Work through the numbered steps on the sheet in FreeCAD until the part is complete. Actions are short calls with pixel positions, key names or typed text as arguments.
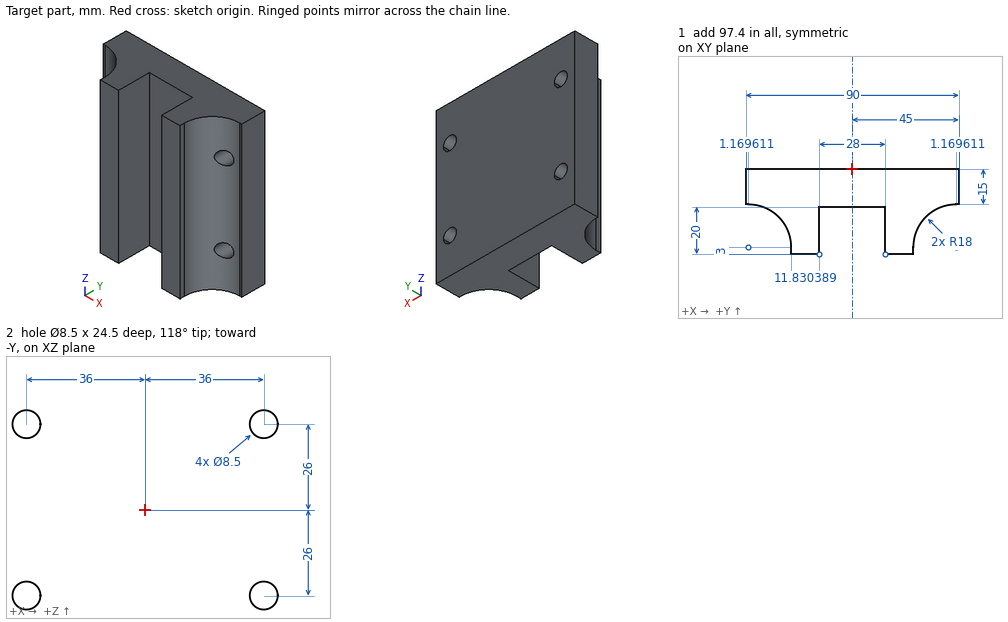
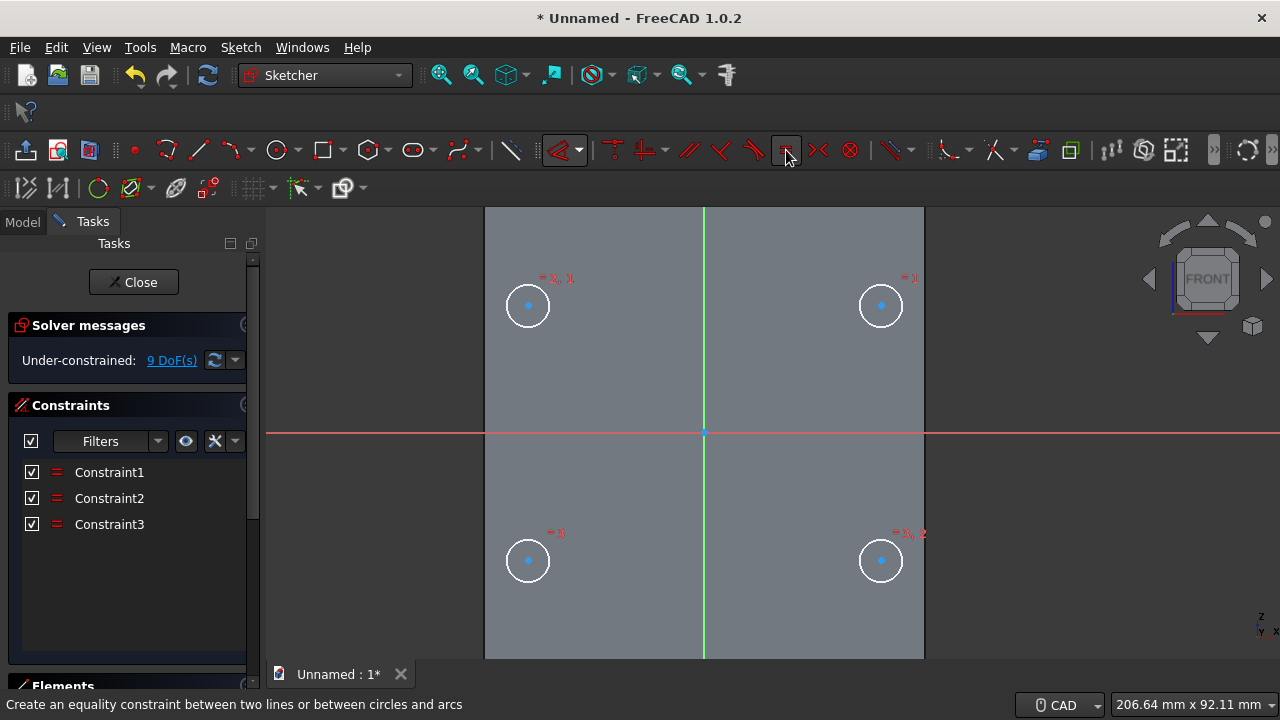
click(881, 306)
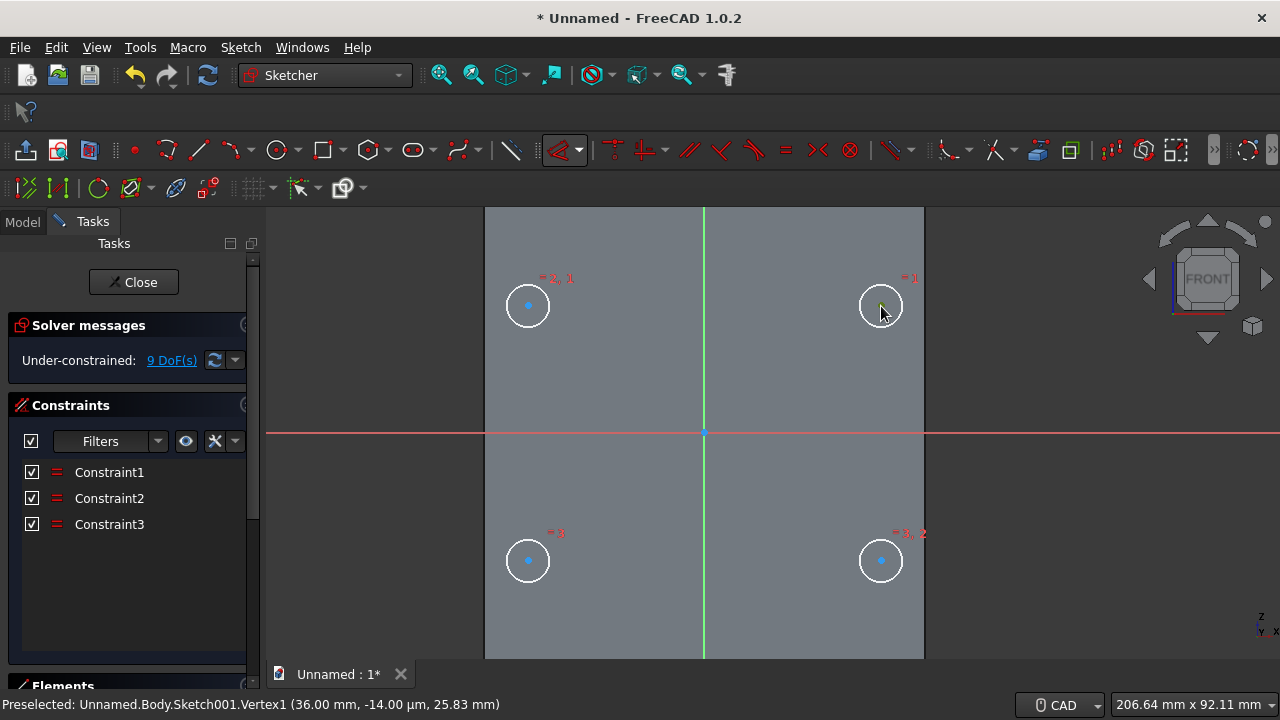
click(528, 306)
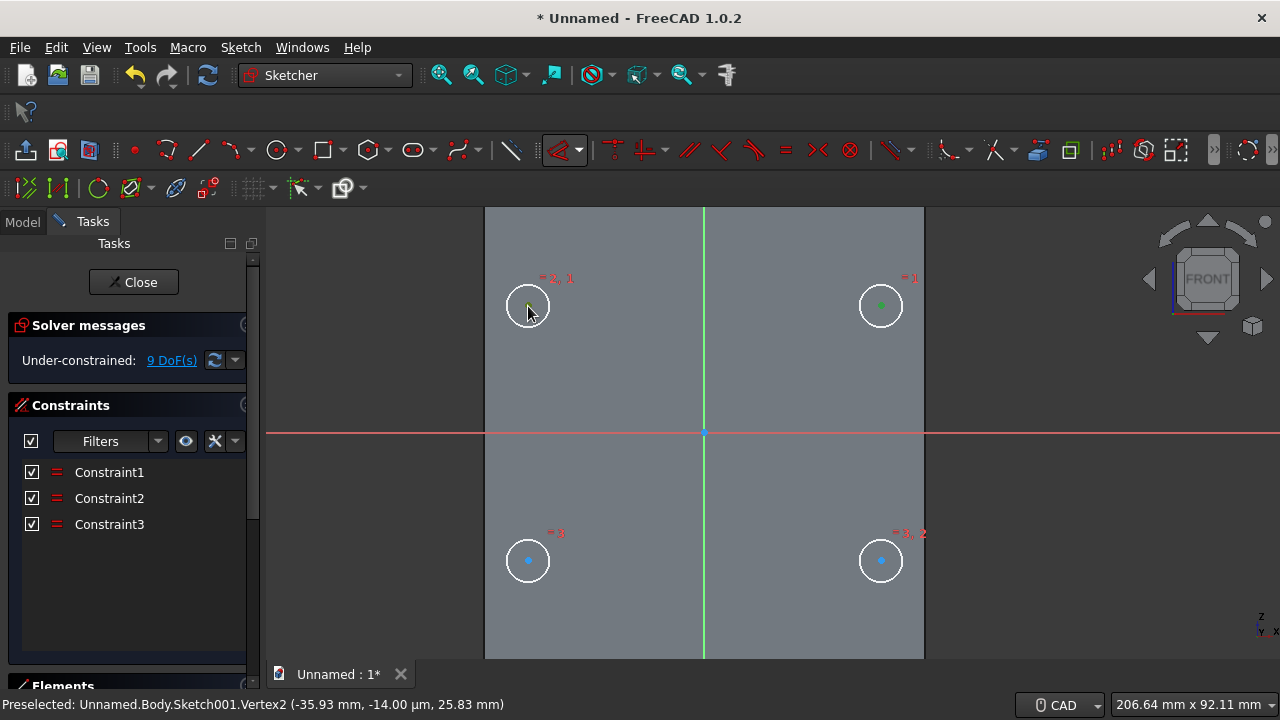
key(h)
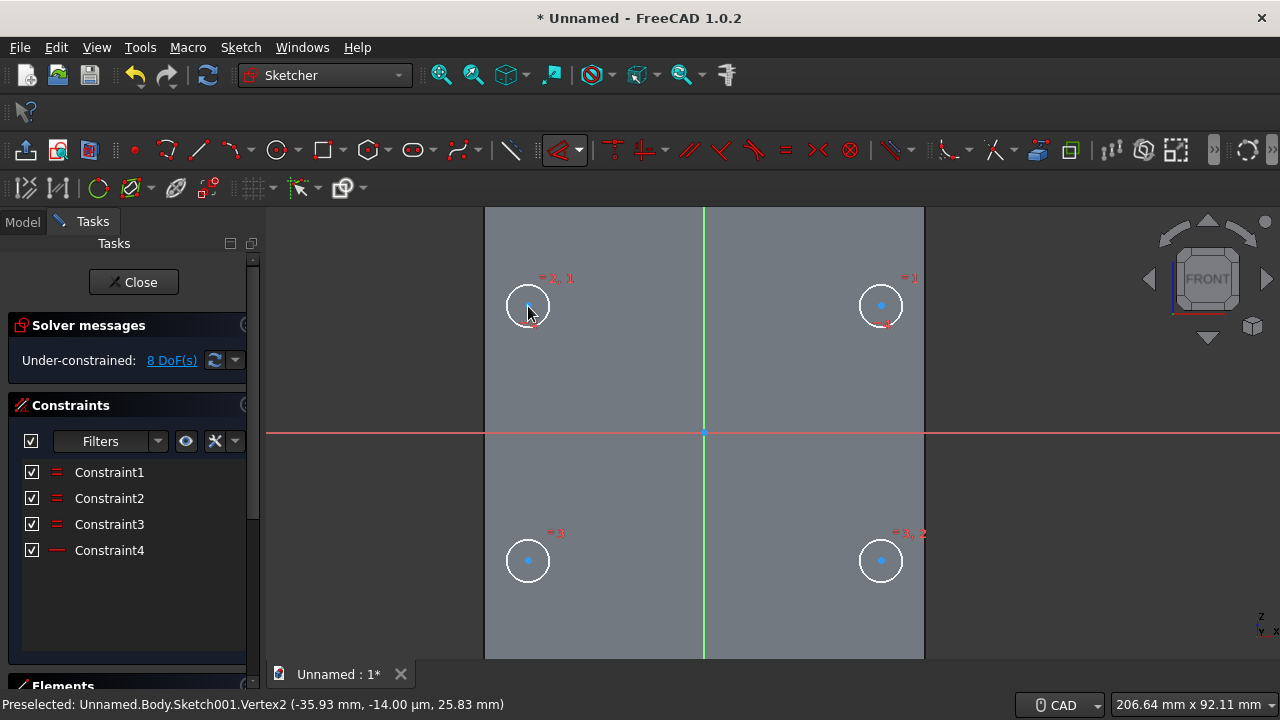
click(881, 306)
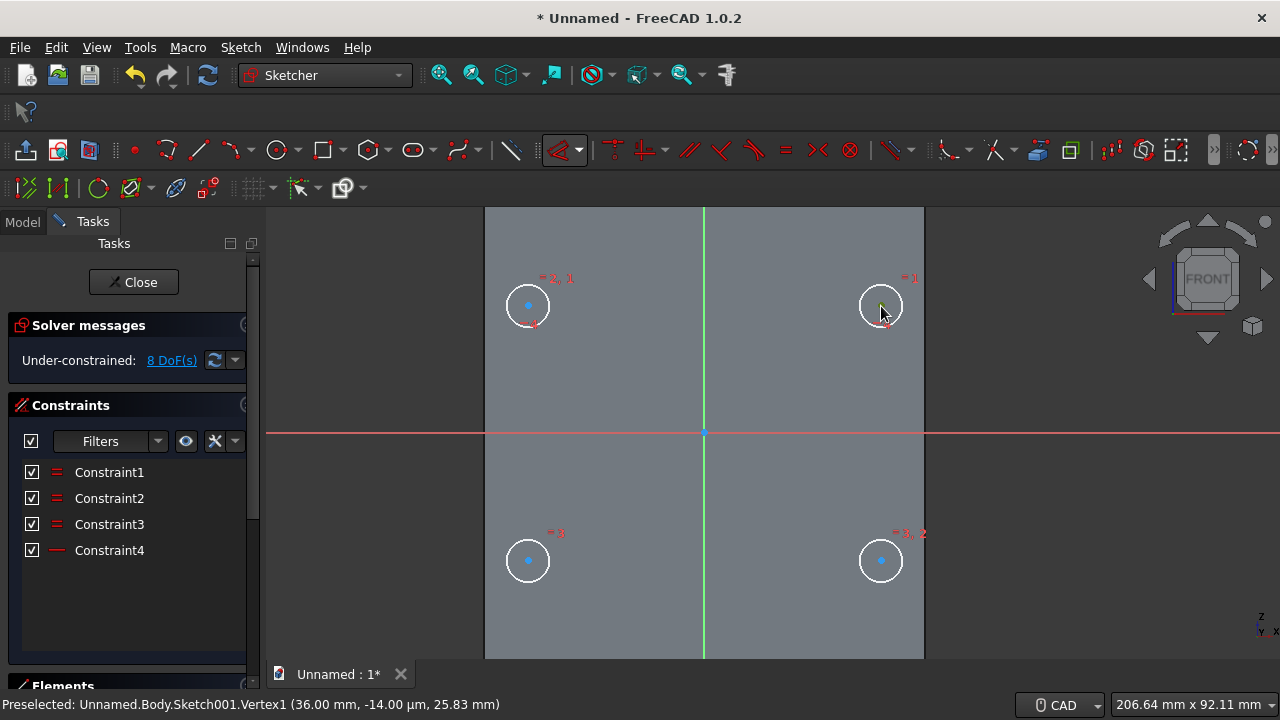
click(881, 561)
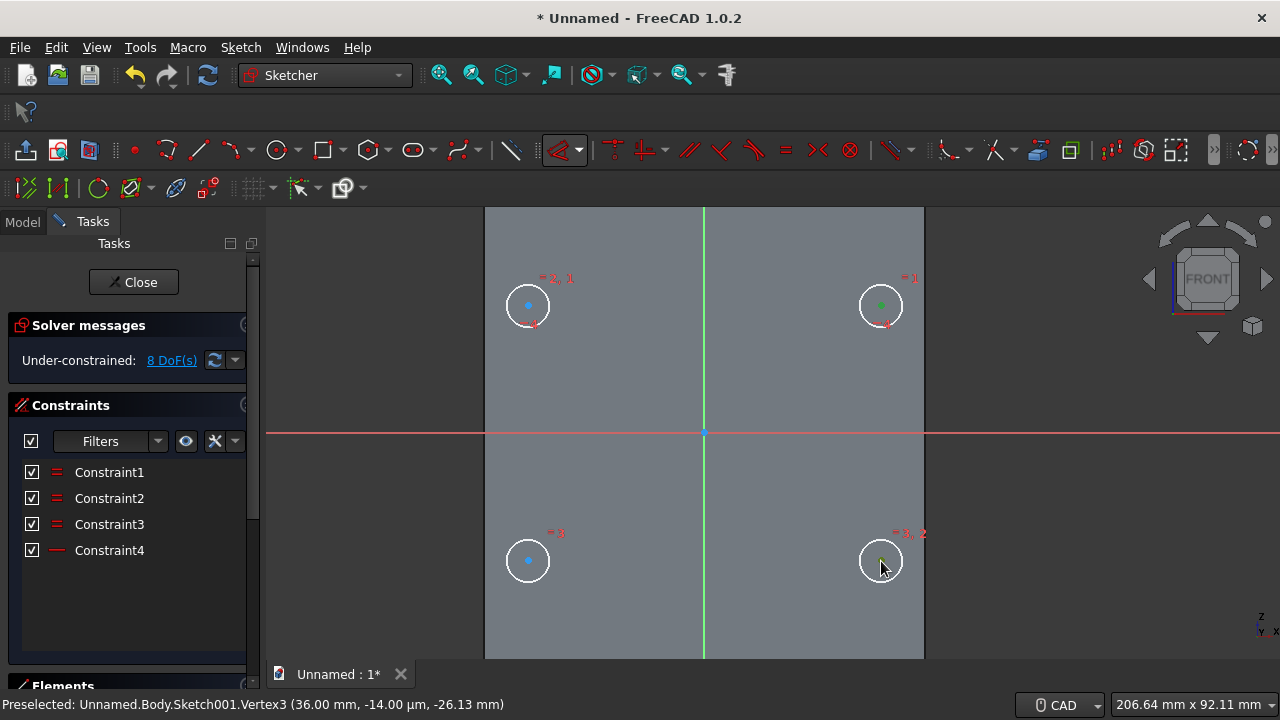
key(v)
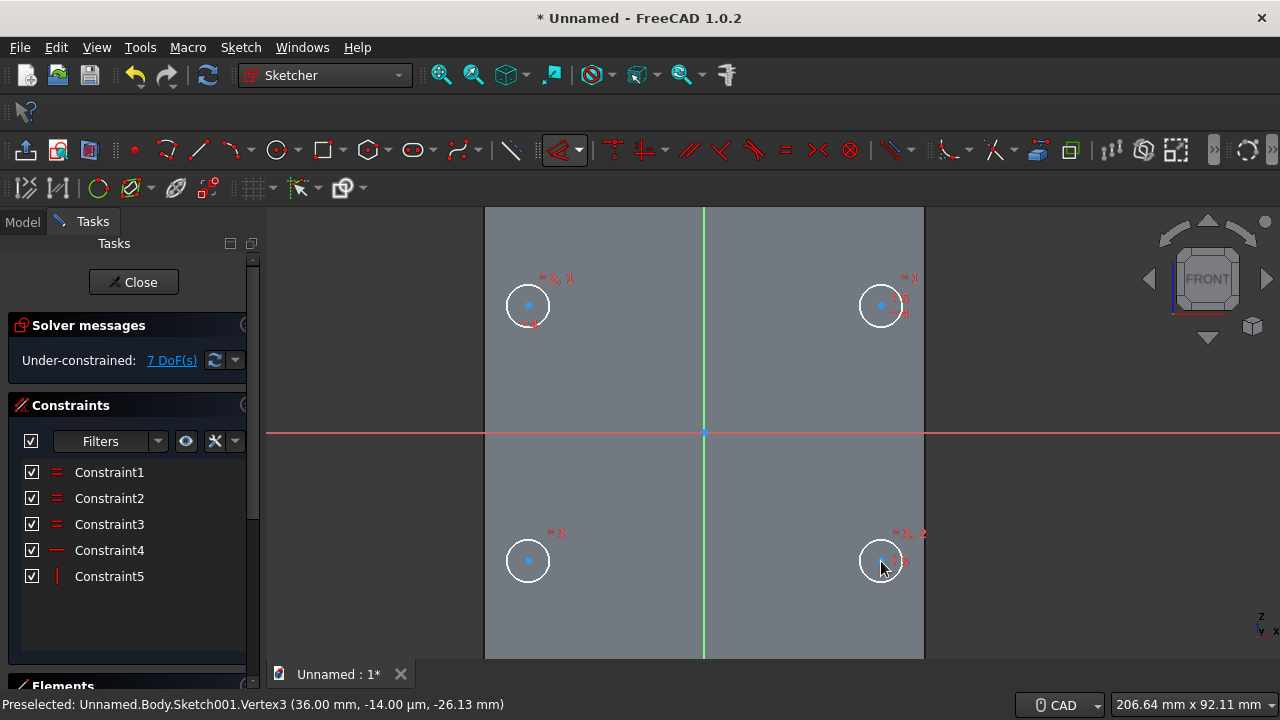
click(528, 306)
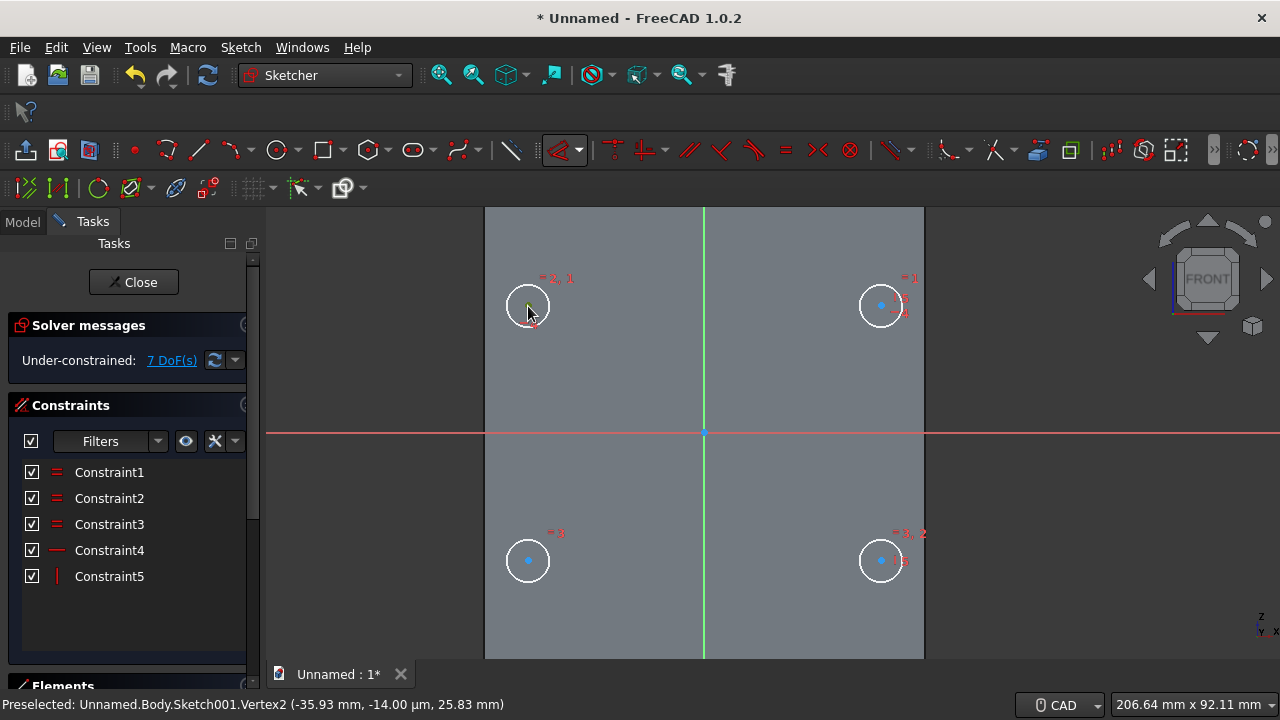
click(528, 561)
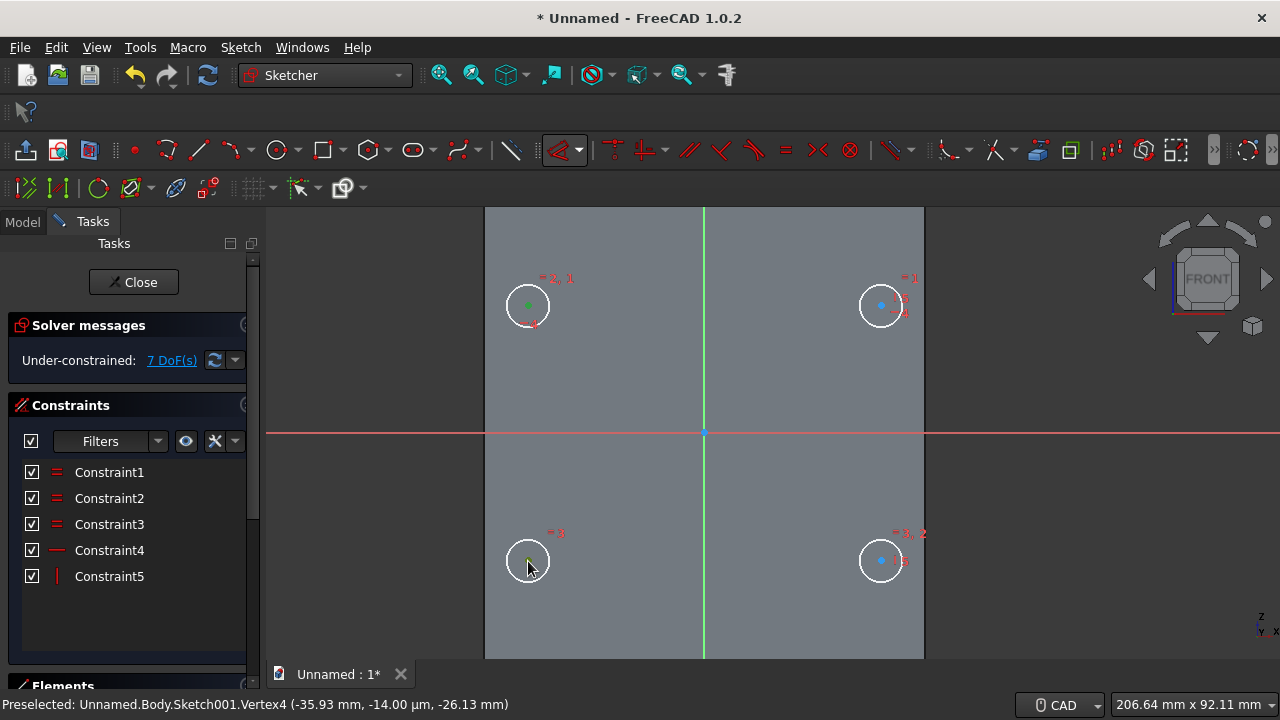
key(v)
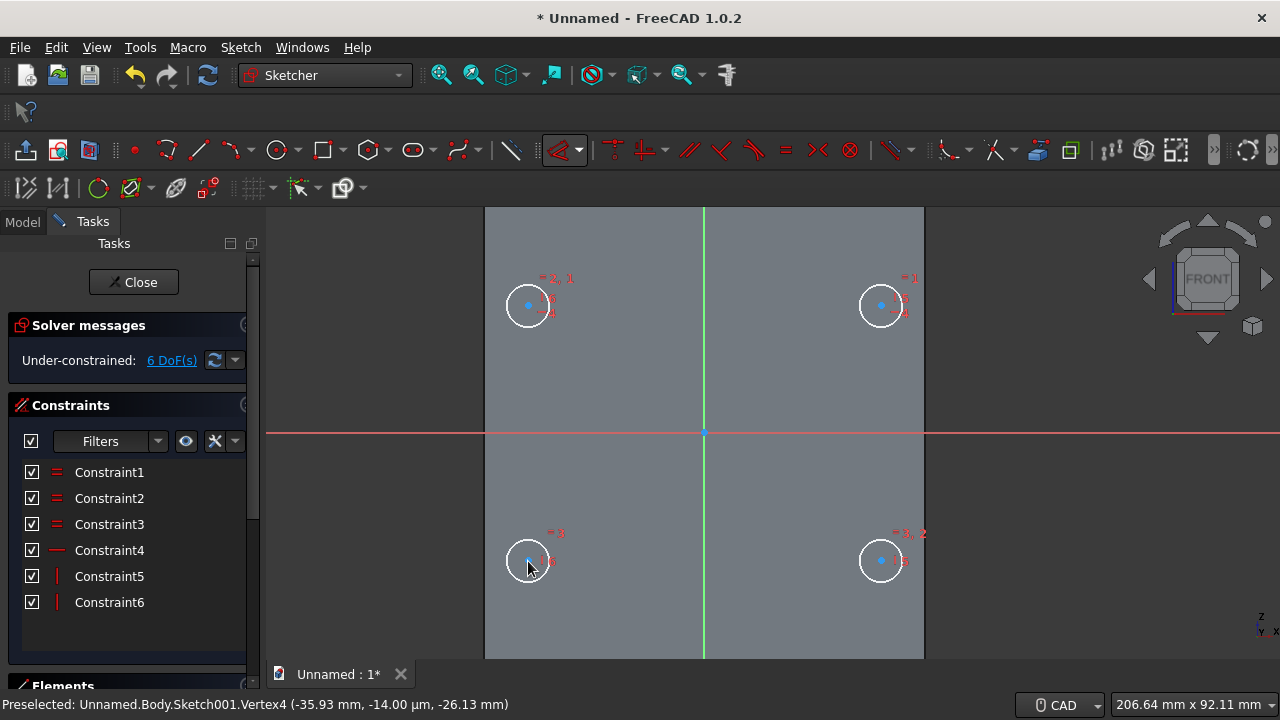
click(881, 561)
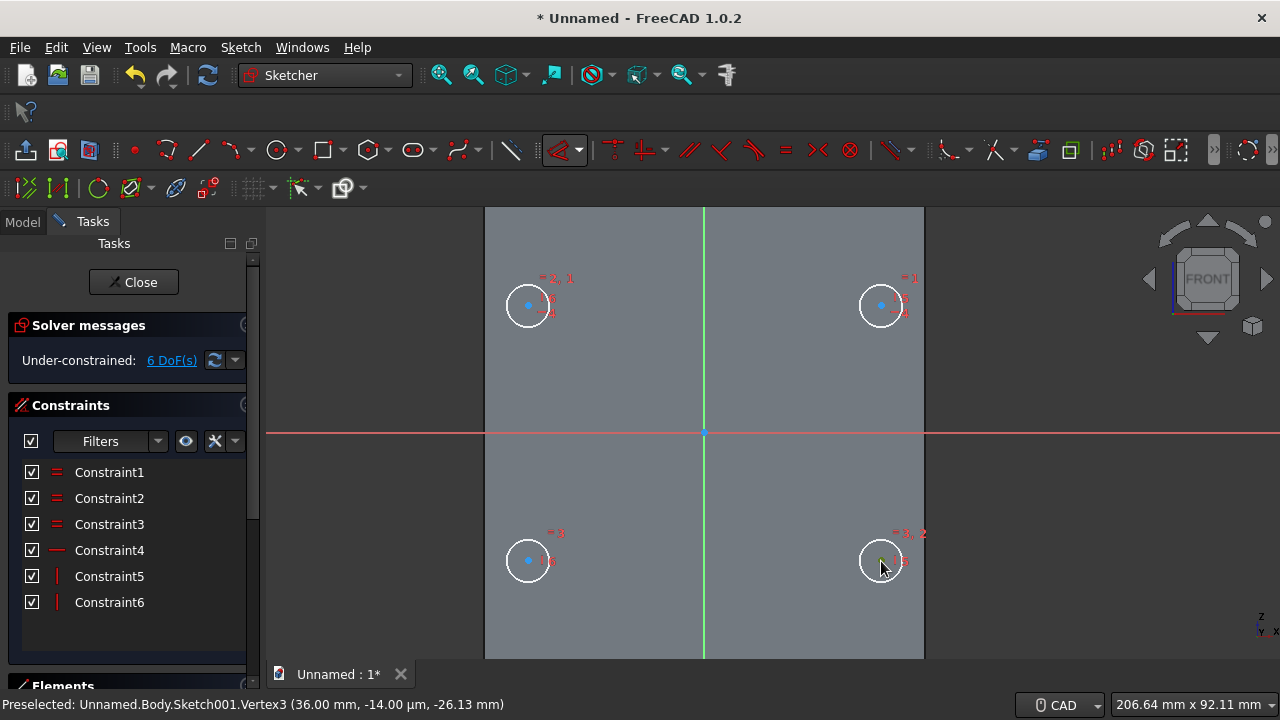
click(528, 561)